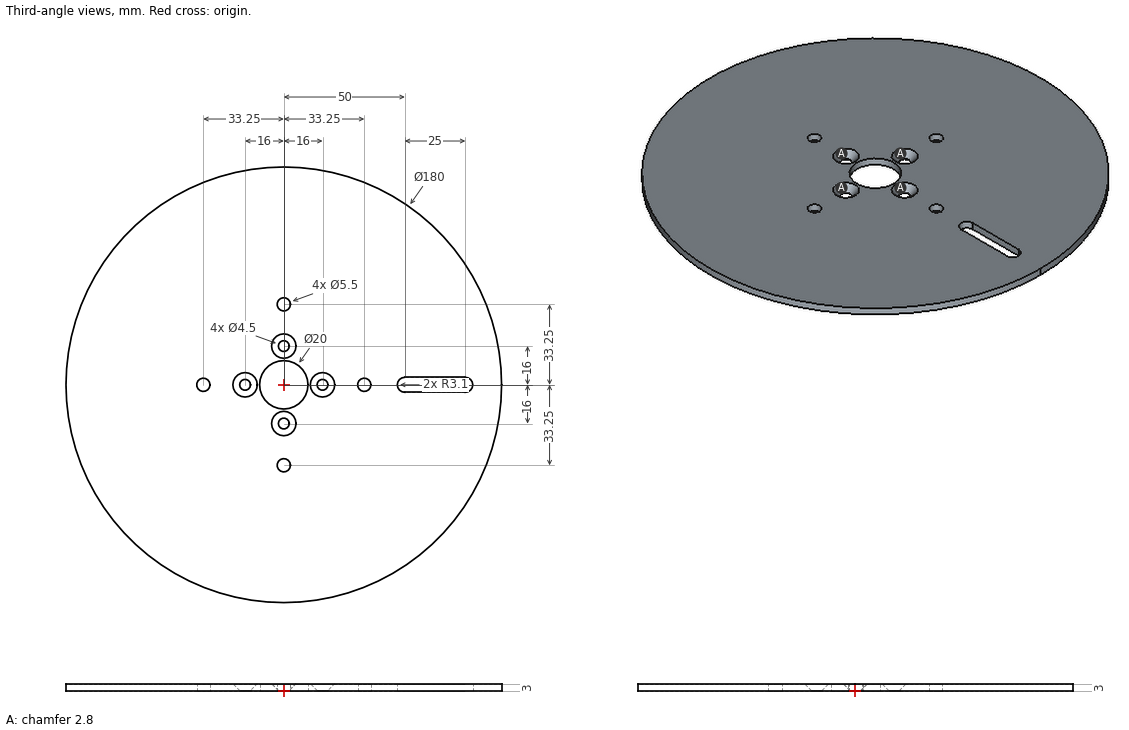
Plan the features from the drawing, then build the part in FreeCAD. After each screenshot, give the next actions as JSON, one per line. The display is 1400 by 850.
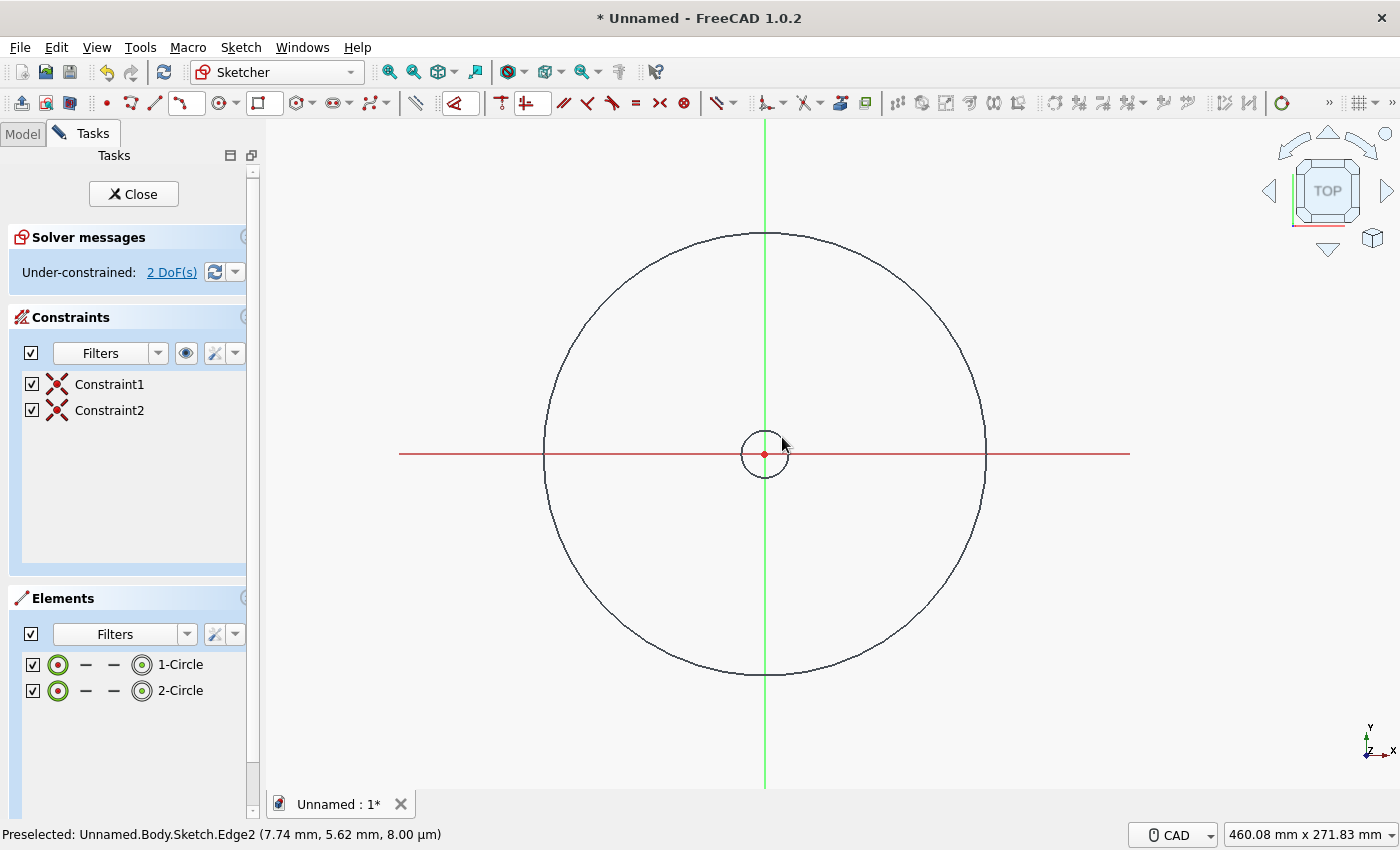
{"action": "left_click", "coordinate": [454, 104]}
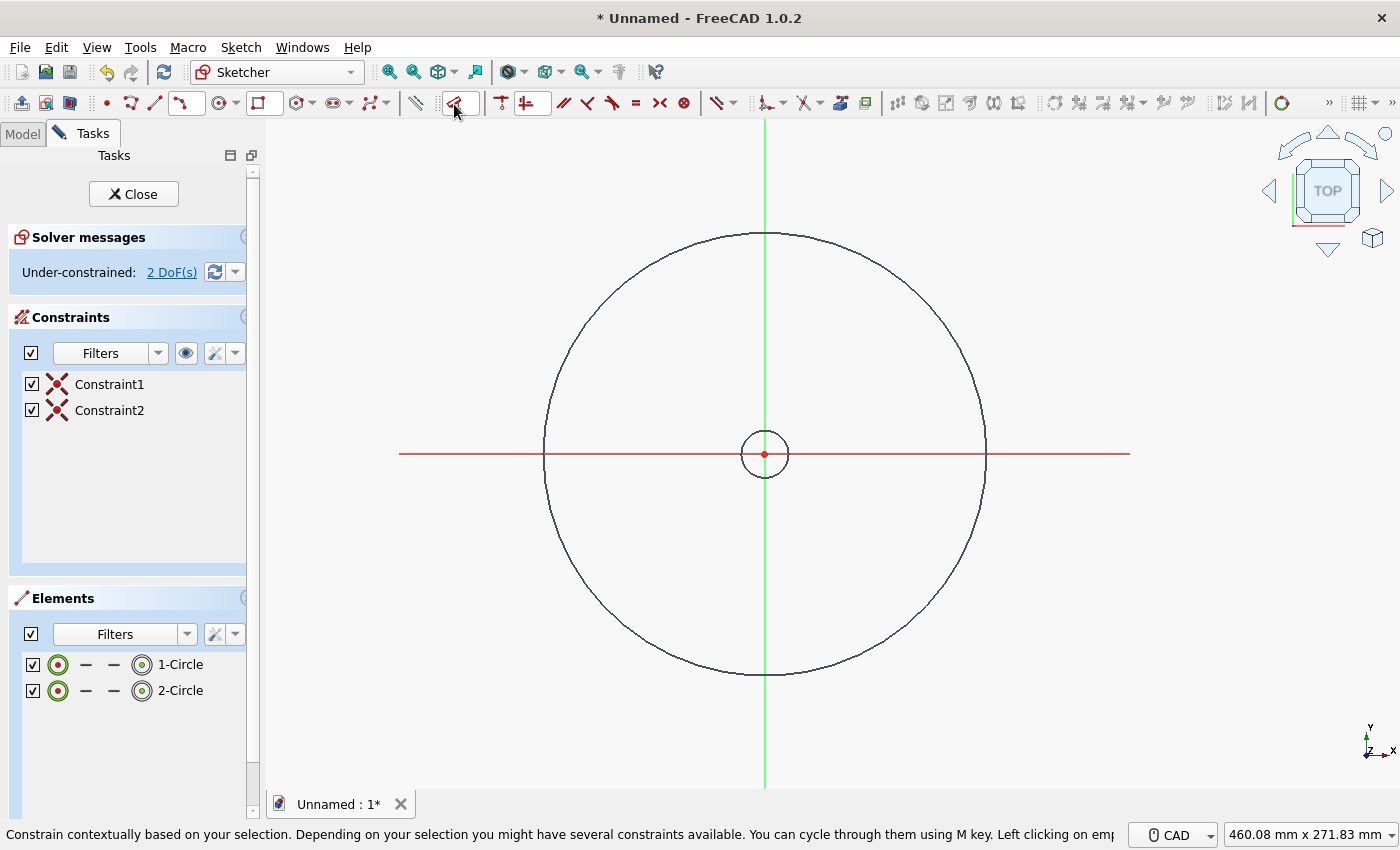
{"action": "left_click", "coordinate": [921, 297]}
{"action": "left_click", "coordinate": [944, 274]}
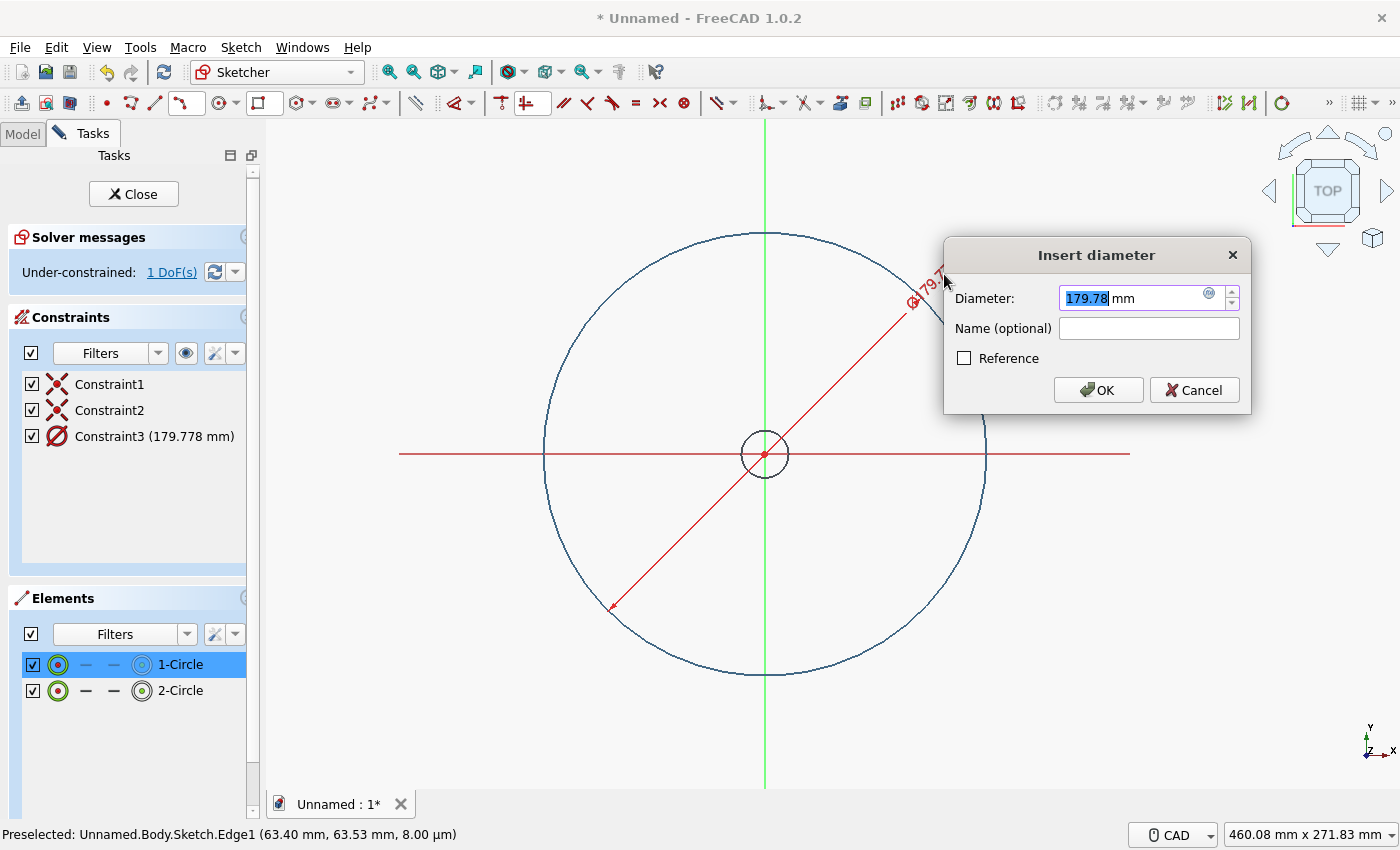
{"action": "type", "text": "180"}
{"action": "key", "text": "Return"}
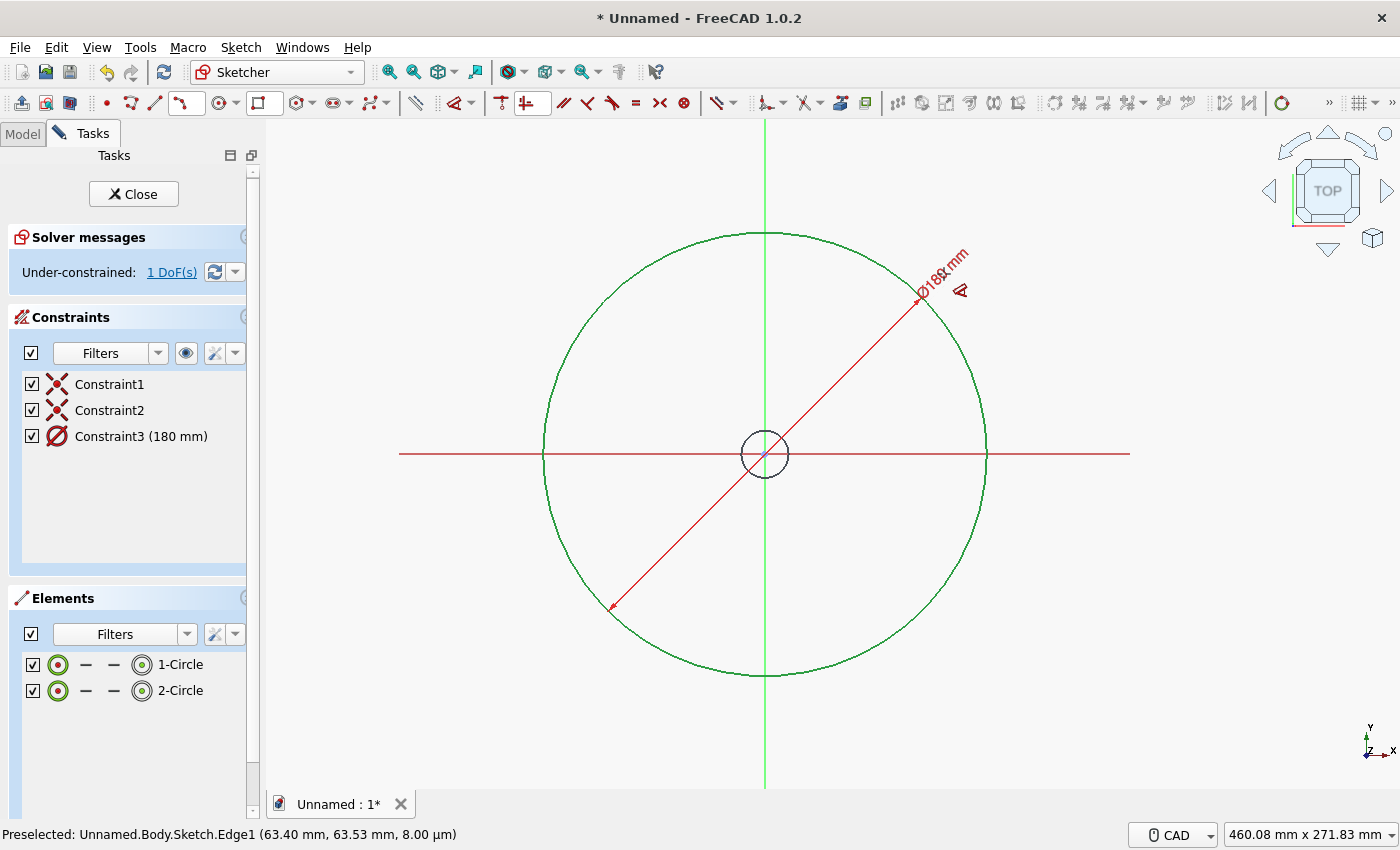
{"action": "left_click", "coordinate": [782, 438]}
{"action": "left_click", "coordinate": [805, 416]}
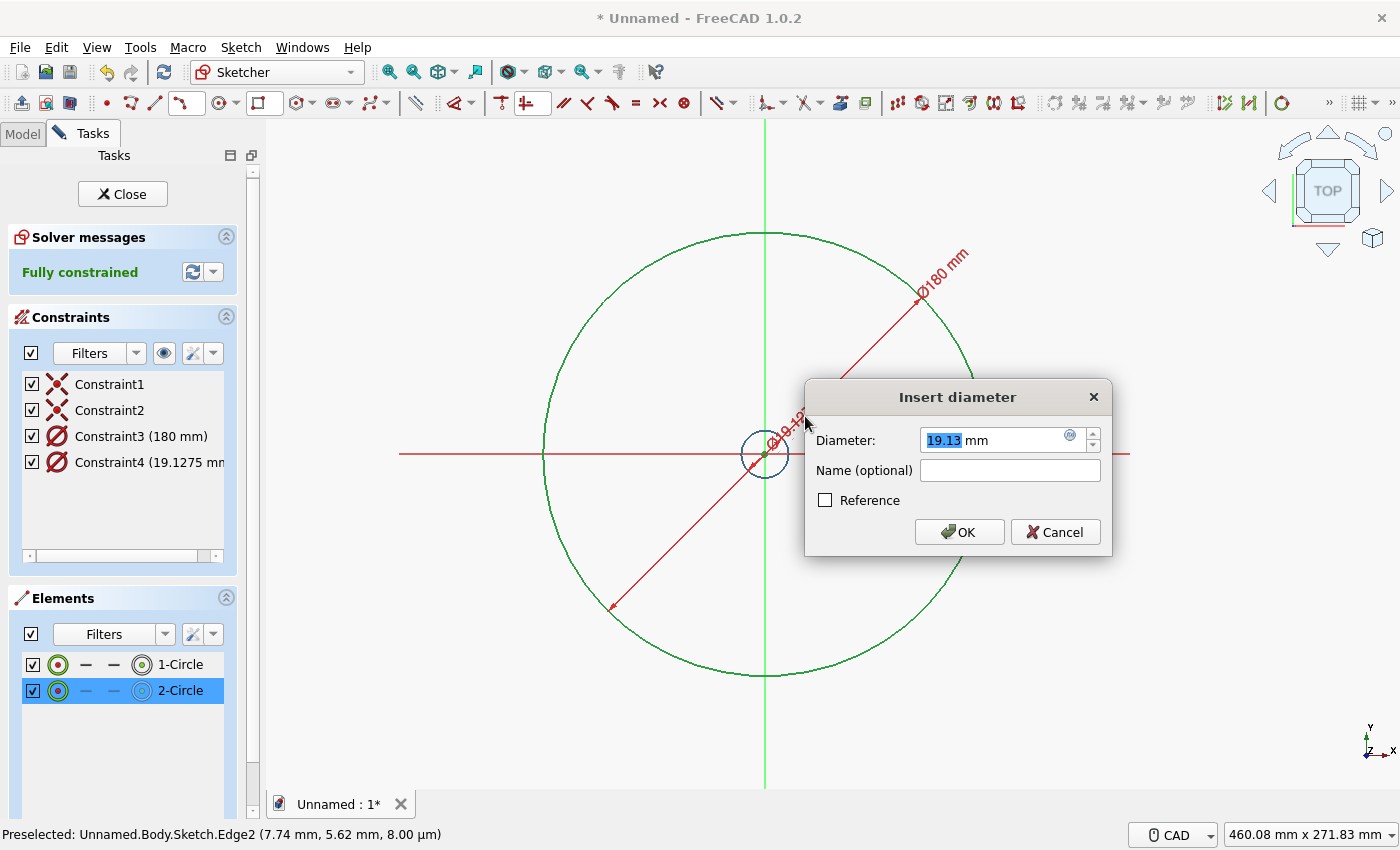
{"action": "type", "text": "20"}
{"action": "key", "text": "Return"}
{"action": "key", "text": "Escape"}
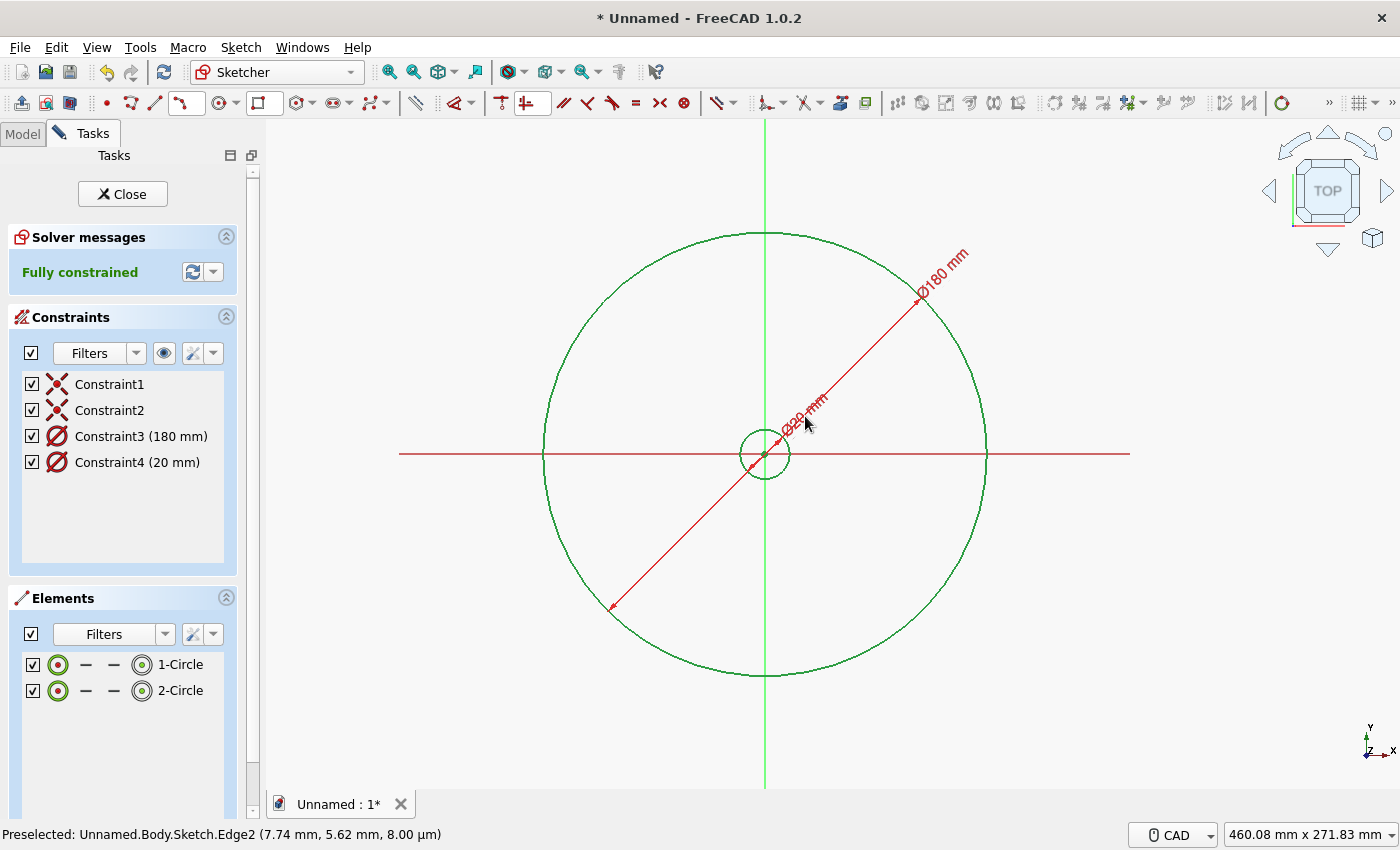
{"action": "left_click", "coordinate": [123, 194]}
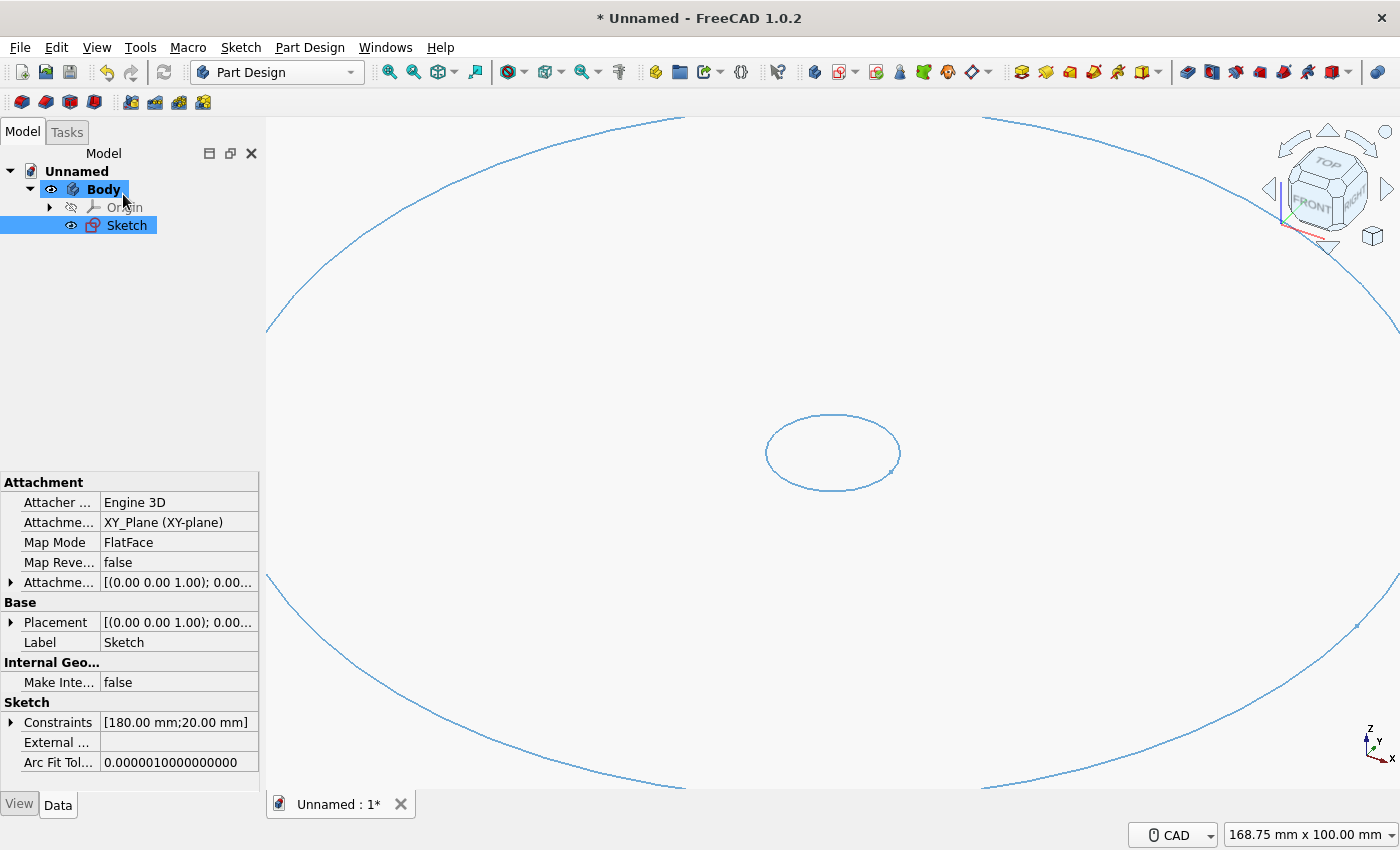
{"action": "left_click", "coordinate": [1022, 72]}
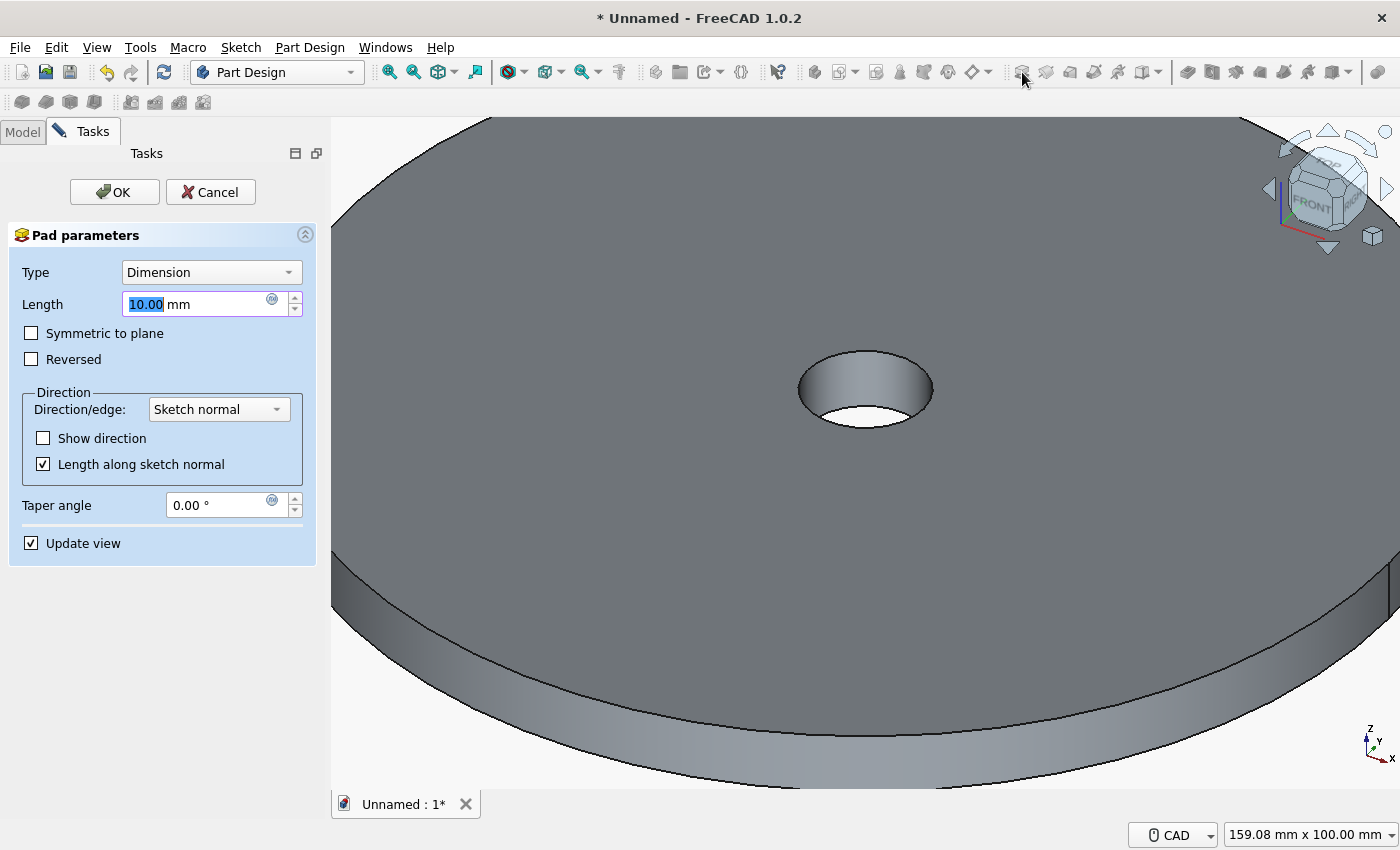
{"action": "type", "text": "3"}
{"action": "key", "text": "Tab"}